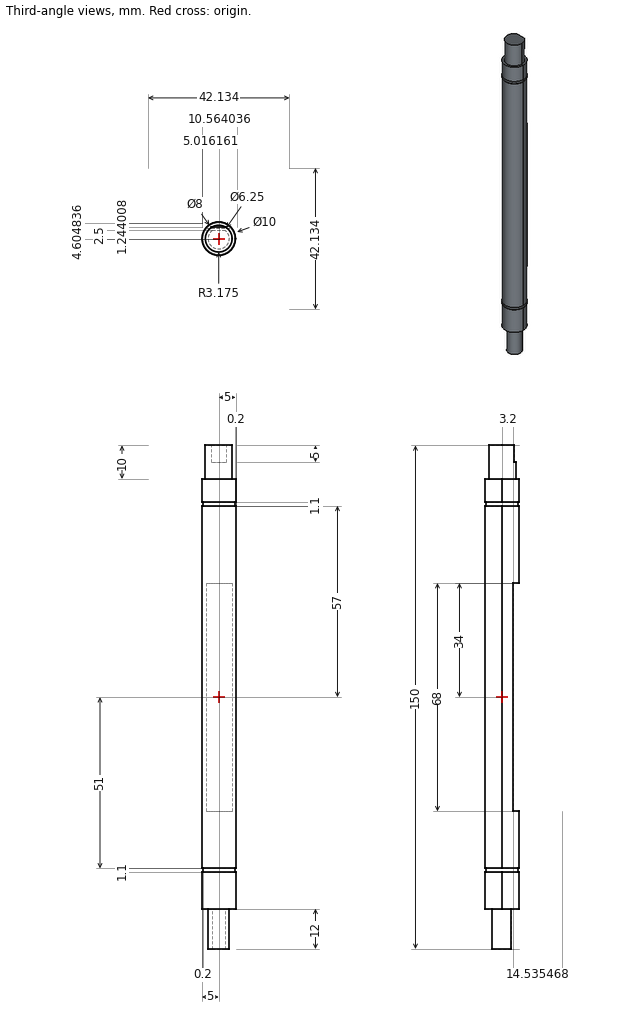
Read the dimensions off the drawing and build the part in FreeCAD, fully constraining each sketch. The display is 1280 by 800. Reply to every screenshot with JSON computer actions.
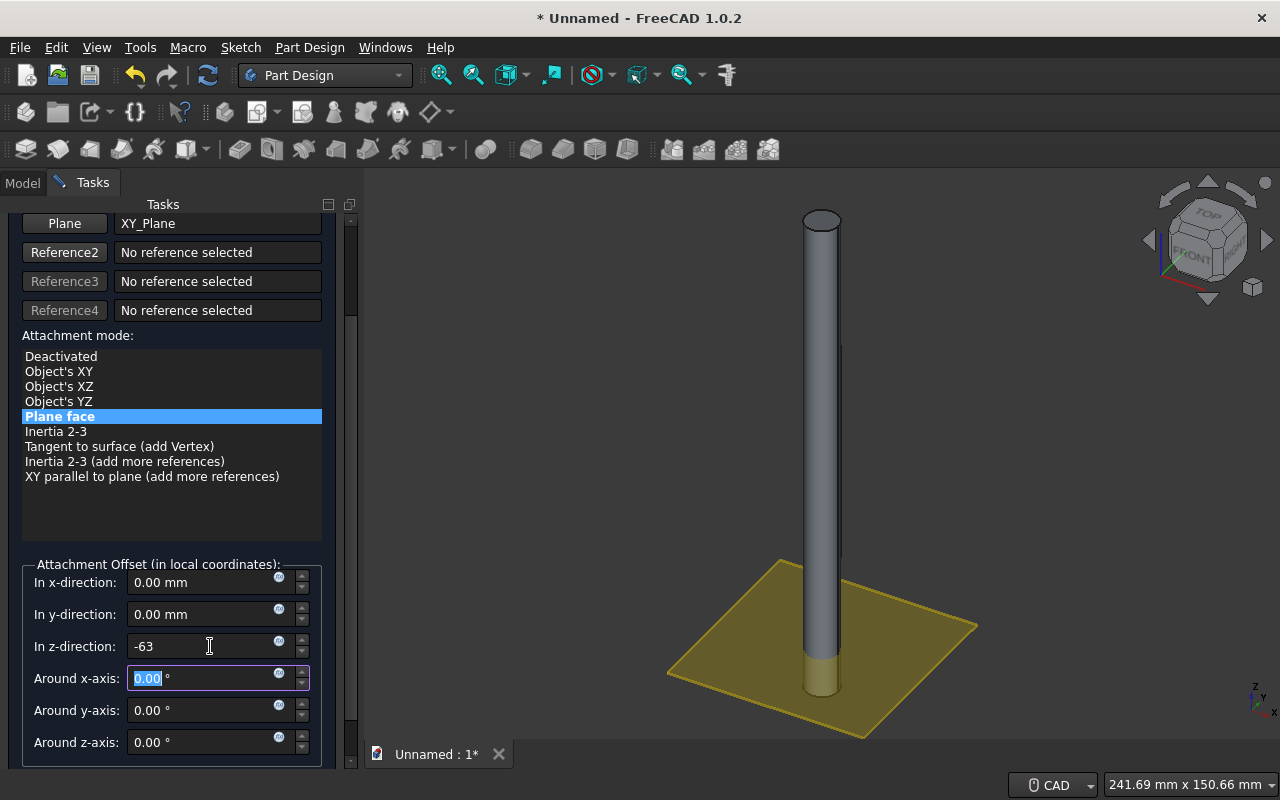
{"action": "scroll", "coordinate": [351, 491], "scroll_direction": "up", "scroll_amount": 3}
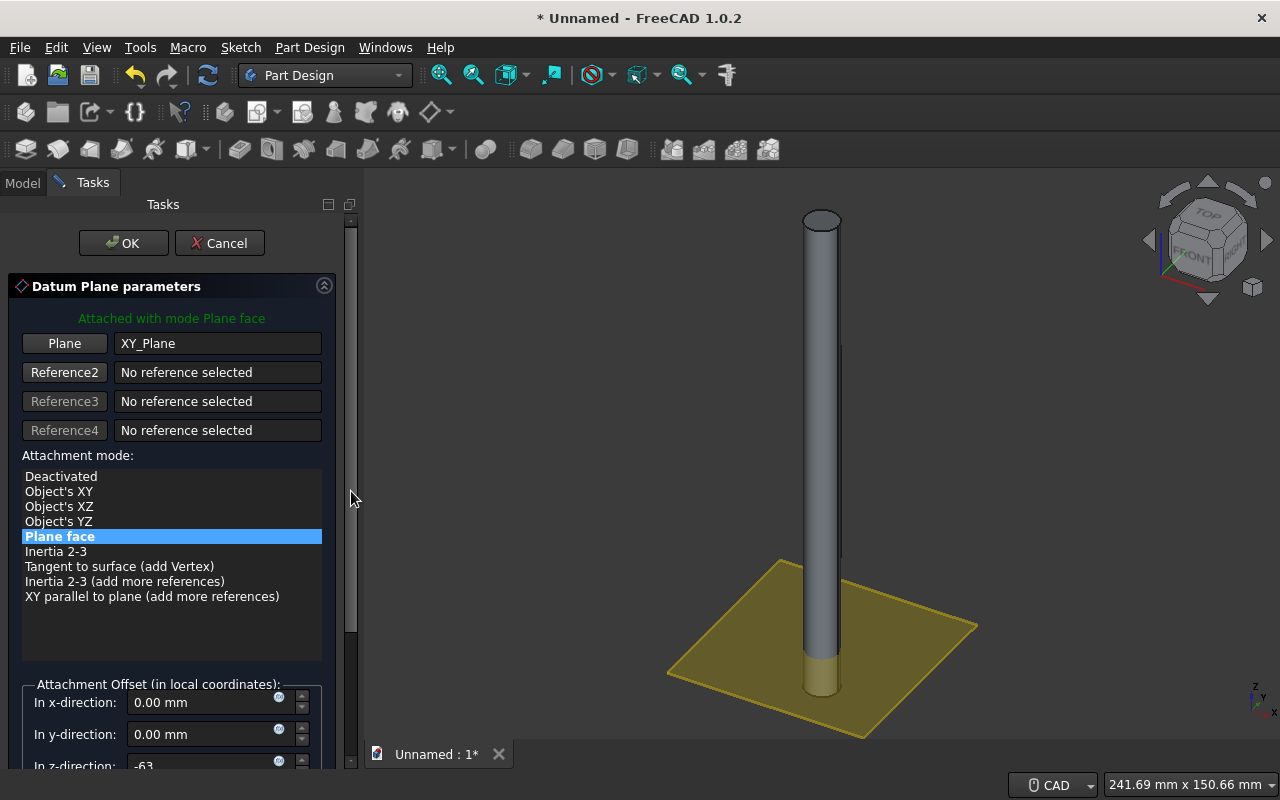
{"action": "left_click", "coordinate": [124, 243]}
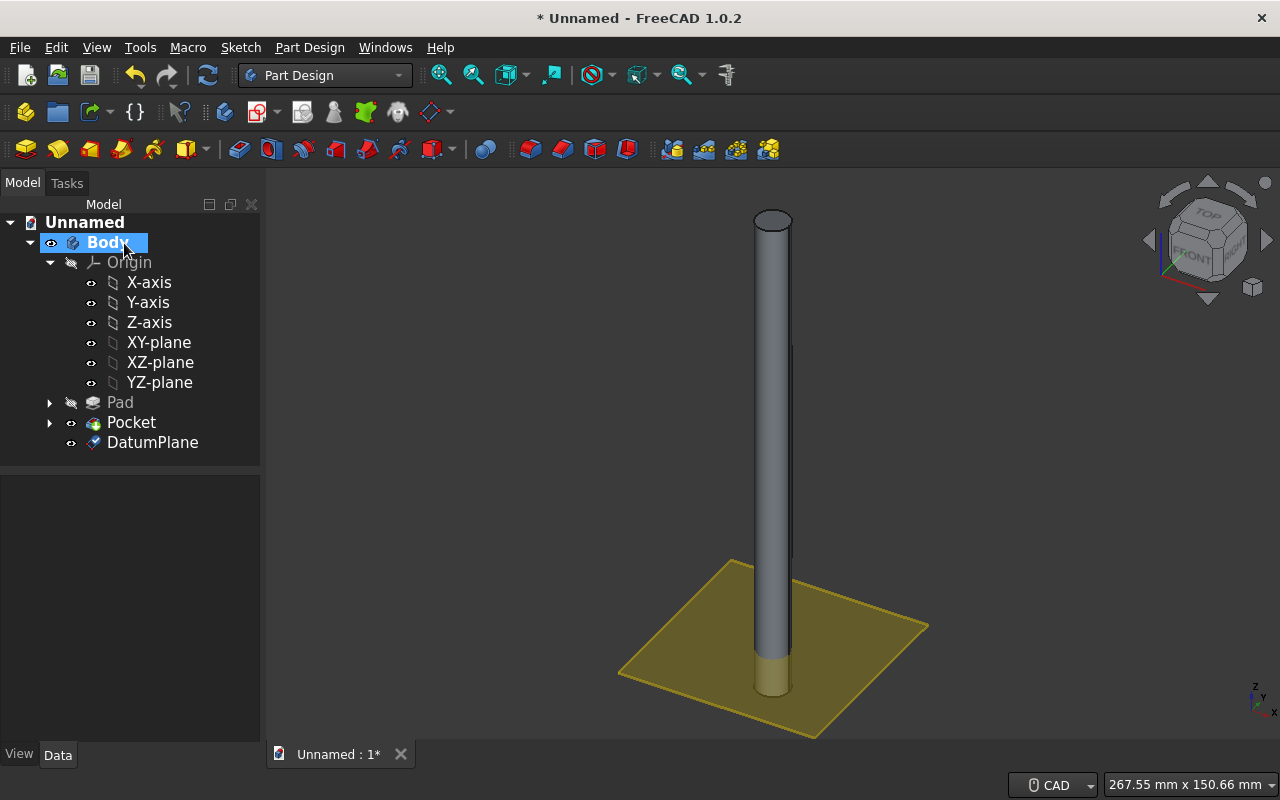
{"action": "left_click", "coordinate": [116, 443]}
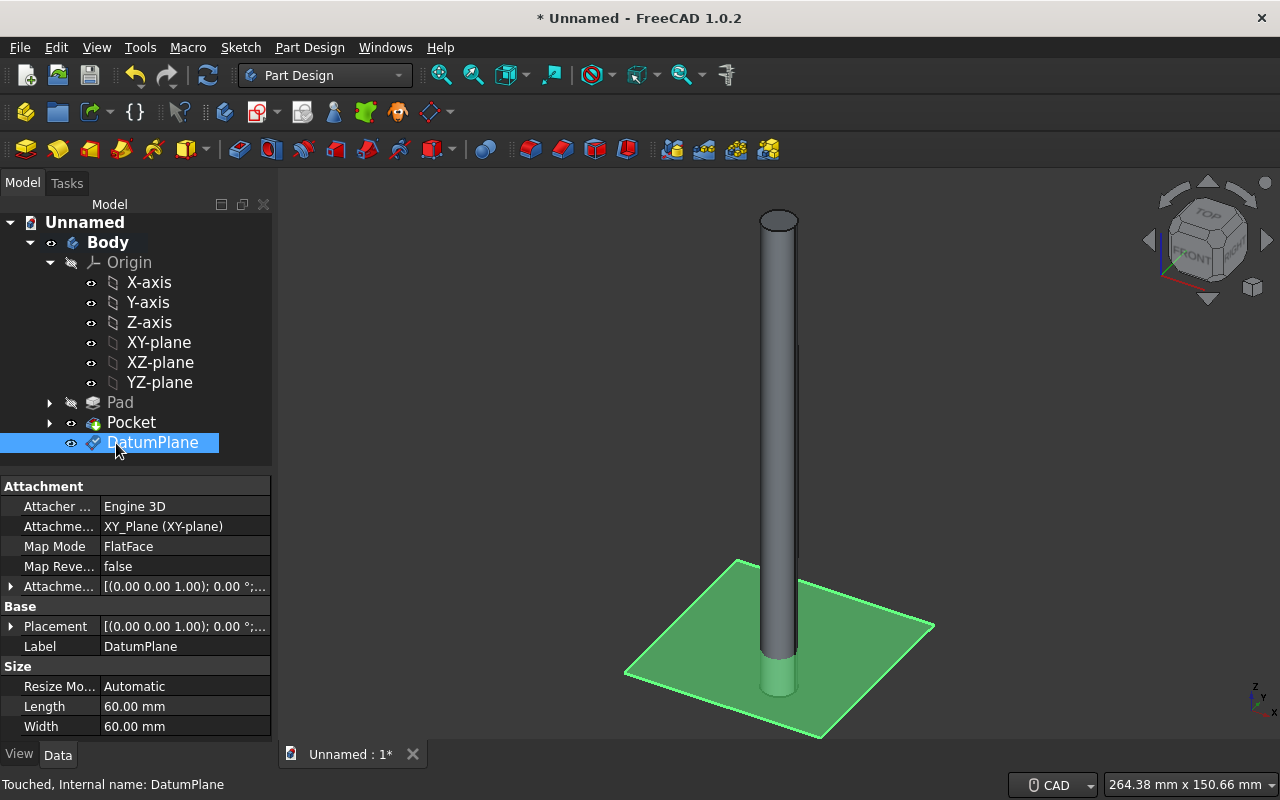
{"action": "left_click", "coordinate": [258, 112]}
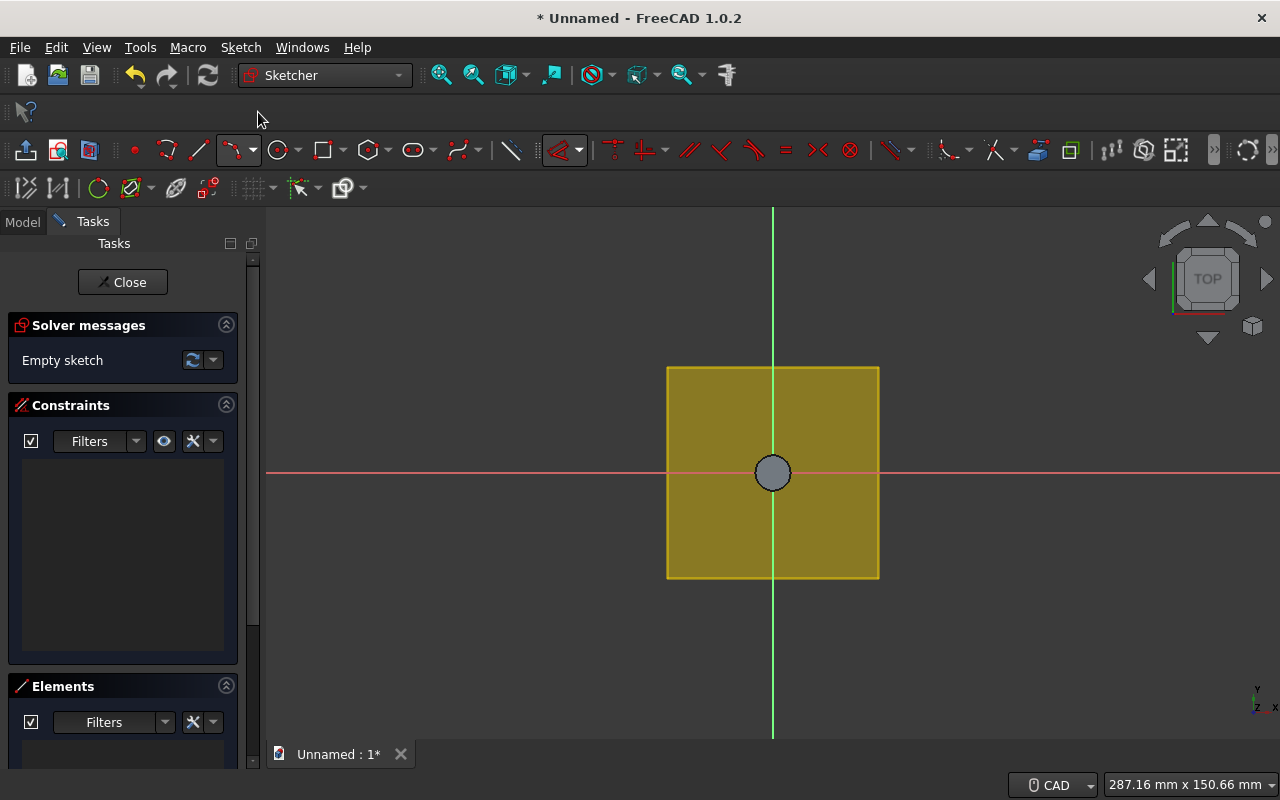
{"action": "left_click", "coordinate": [90, 150]}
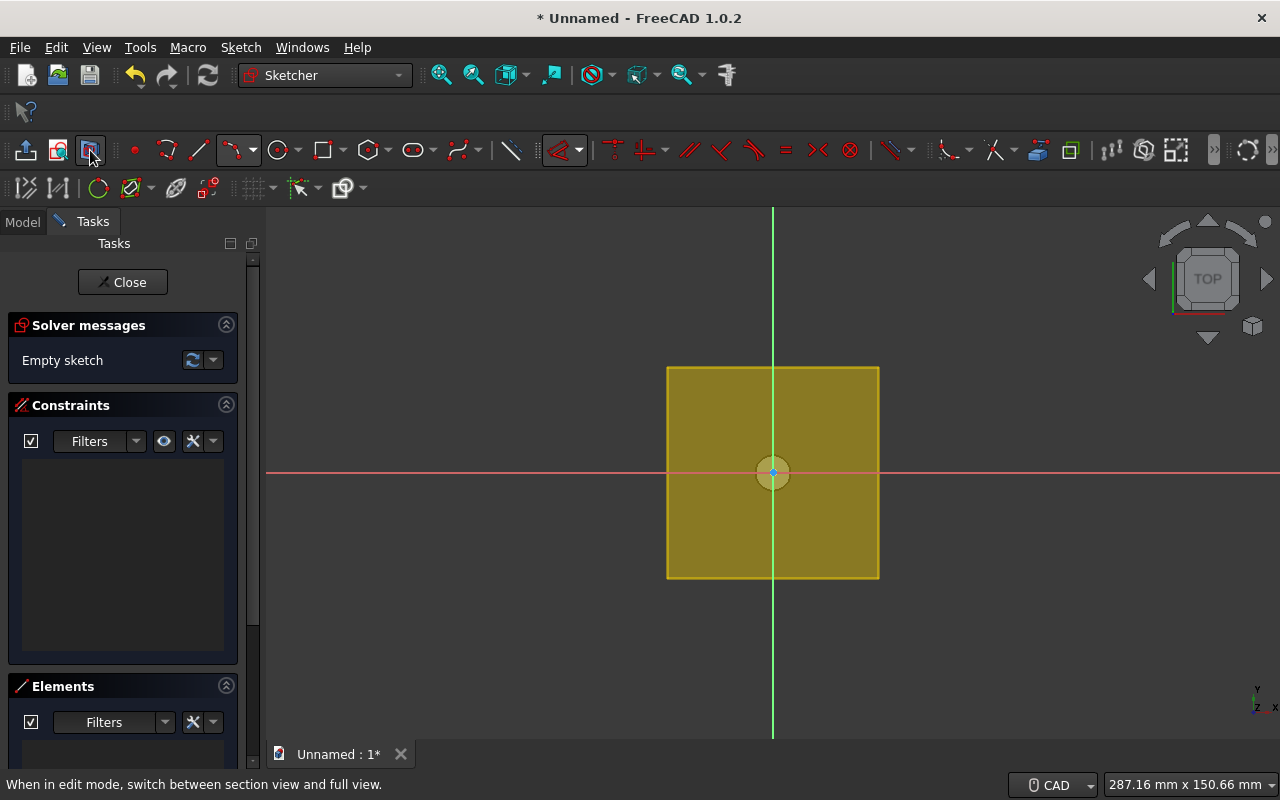
{"action": "scroll", "coordinate": [782, 473], "scroll_direction": "up", "scroll_amount": 11}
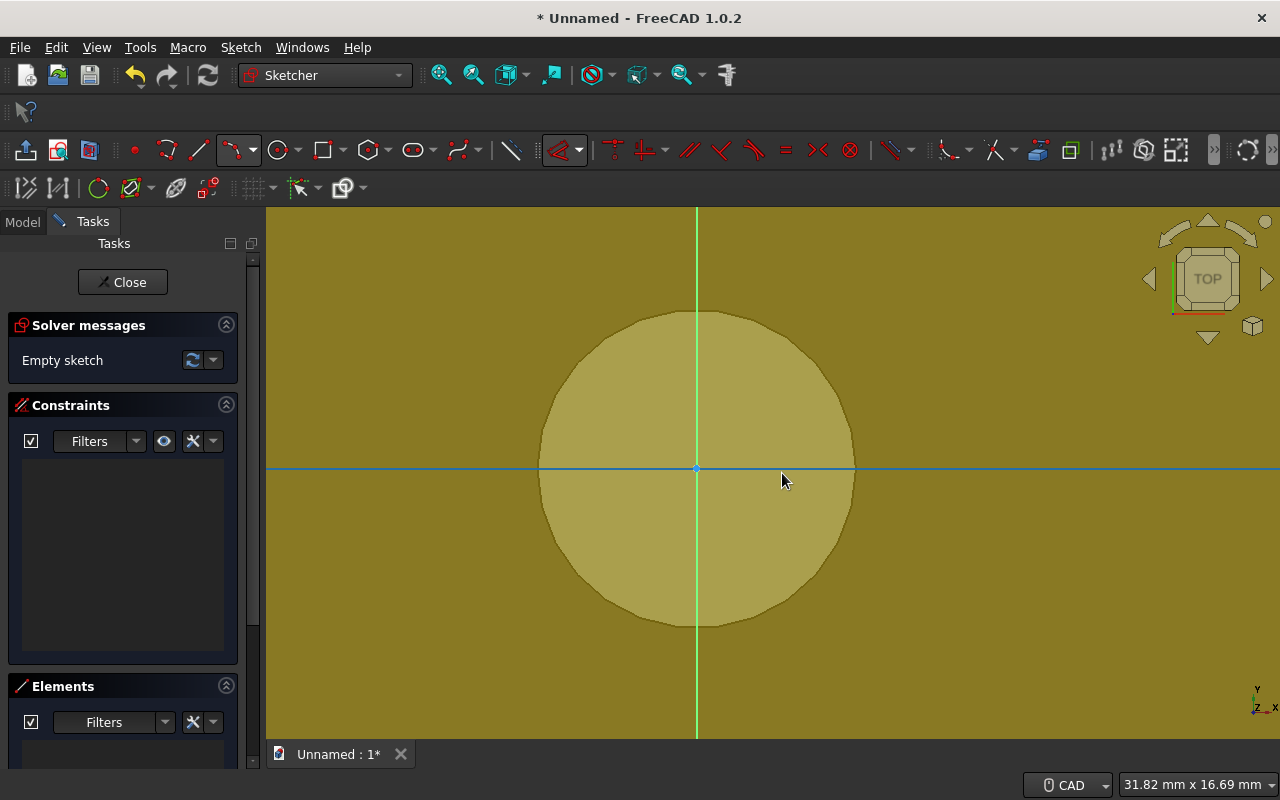
{"action": "left_click", "coordinate": [278, 150]}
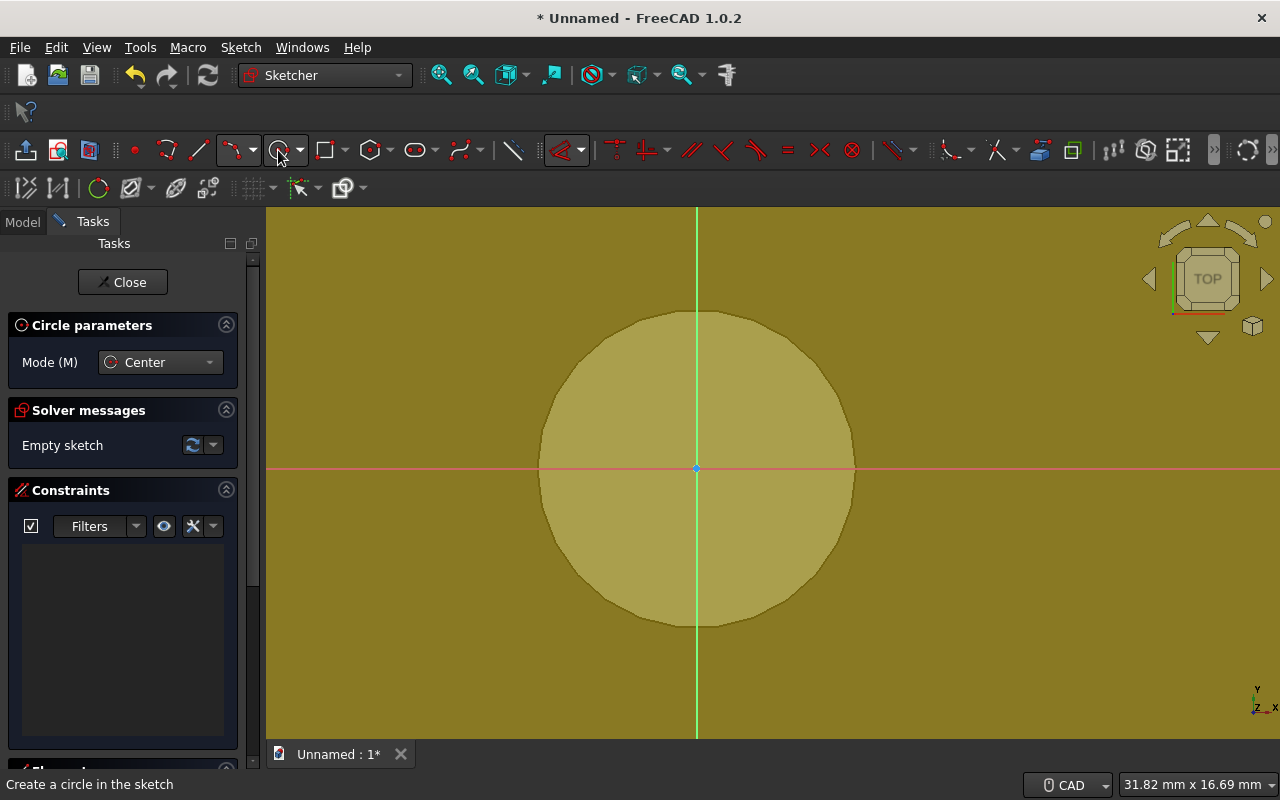
{"action": "left_click", "coordinate": [697, 469]}
{"action": "left_click", "coordinate": [809, 356]}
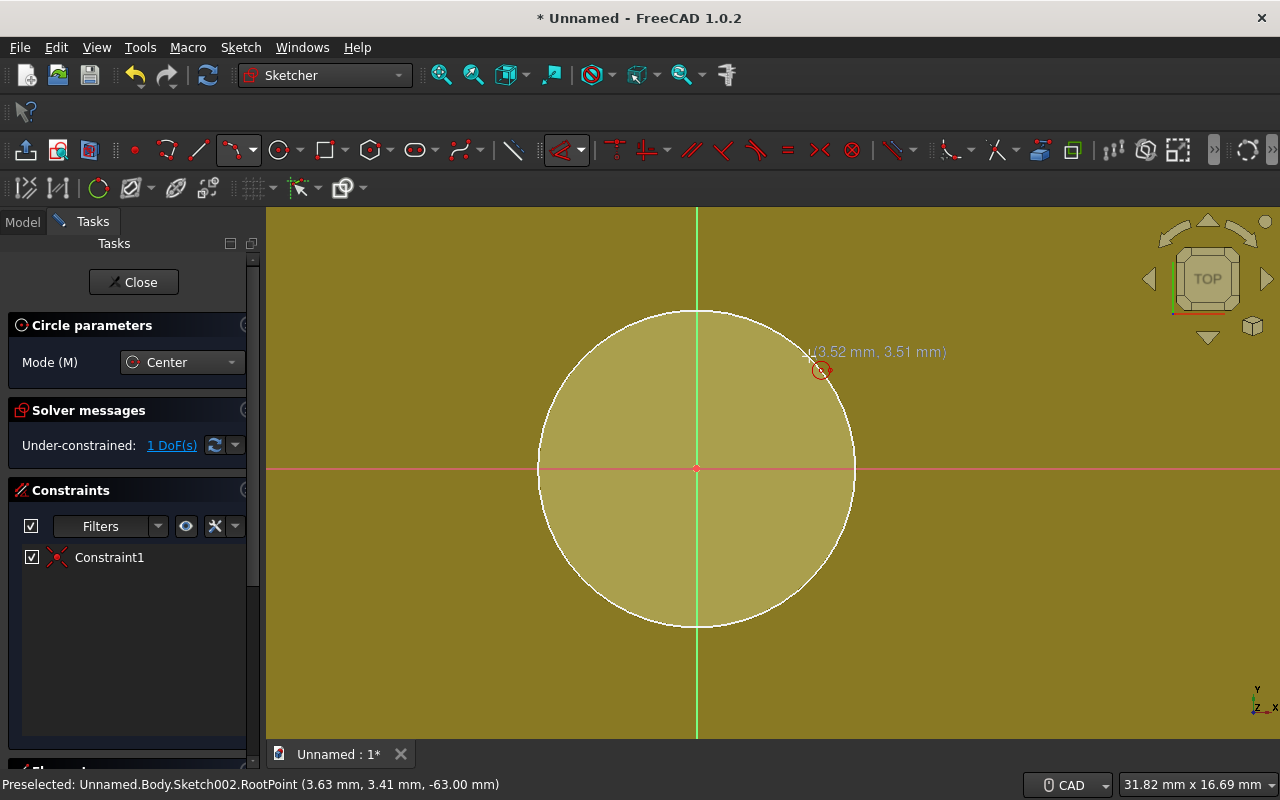
{"action": "left_click", "coordinate": [697, 469]}
{"action": "left_click", "coordinate": [767, 399]}
{"action": "key", "text": "Escape"}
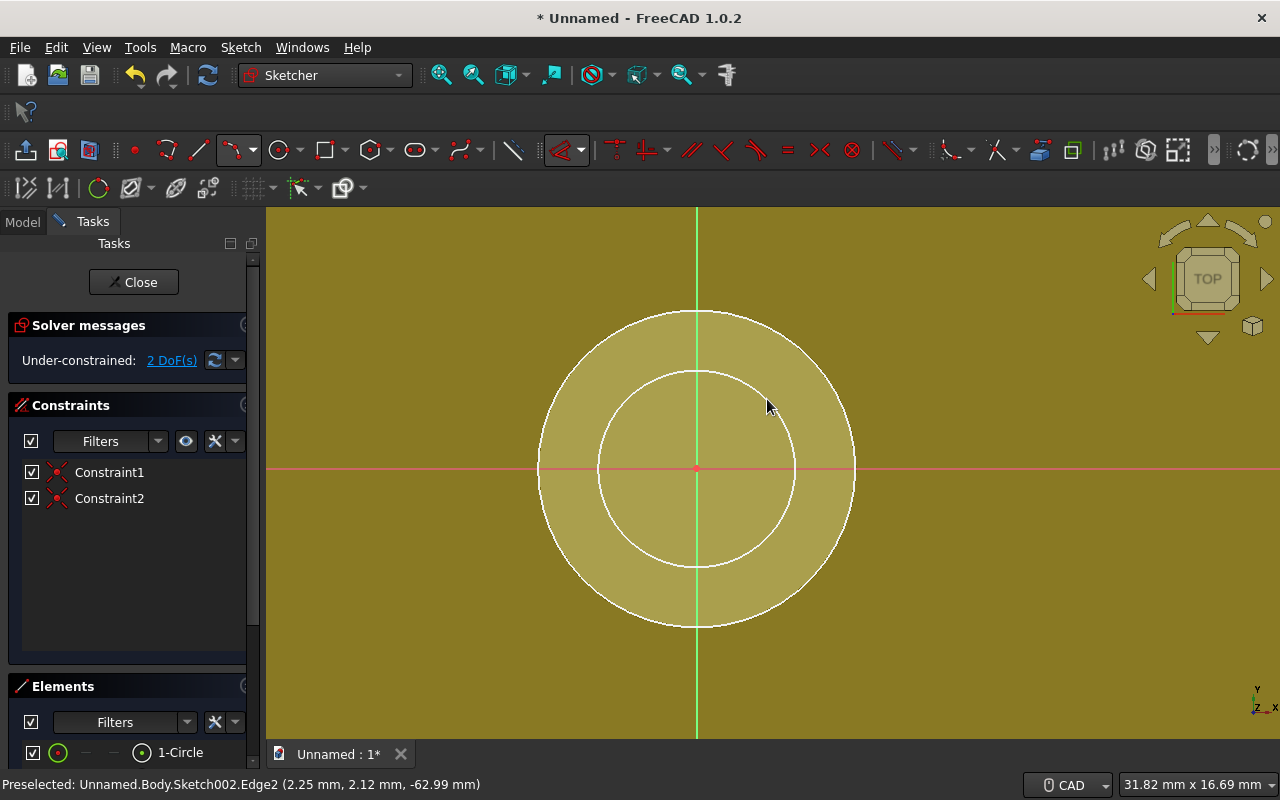
{"action": "left_click", "coordinate": [808, 356]}